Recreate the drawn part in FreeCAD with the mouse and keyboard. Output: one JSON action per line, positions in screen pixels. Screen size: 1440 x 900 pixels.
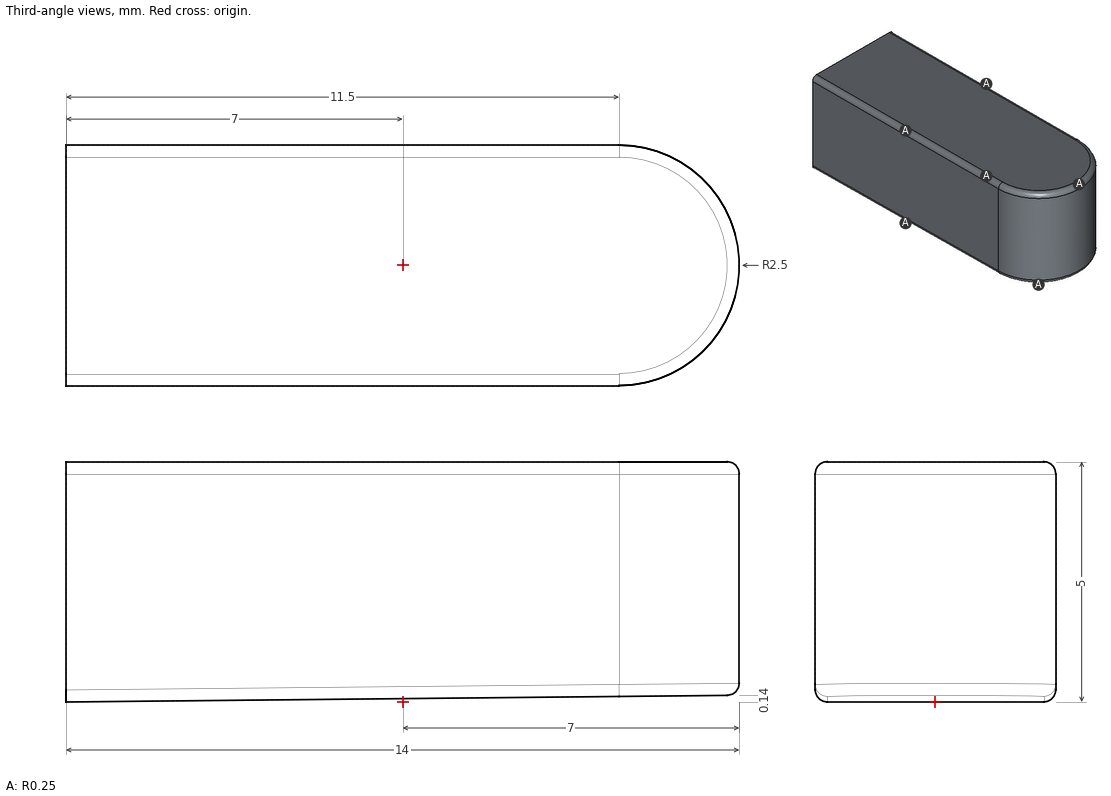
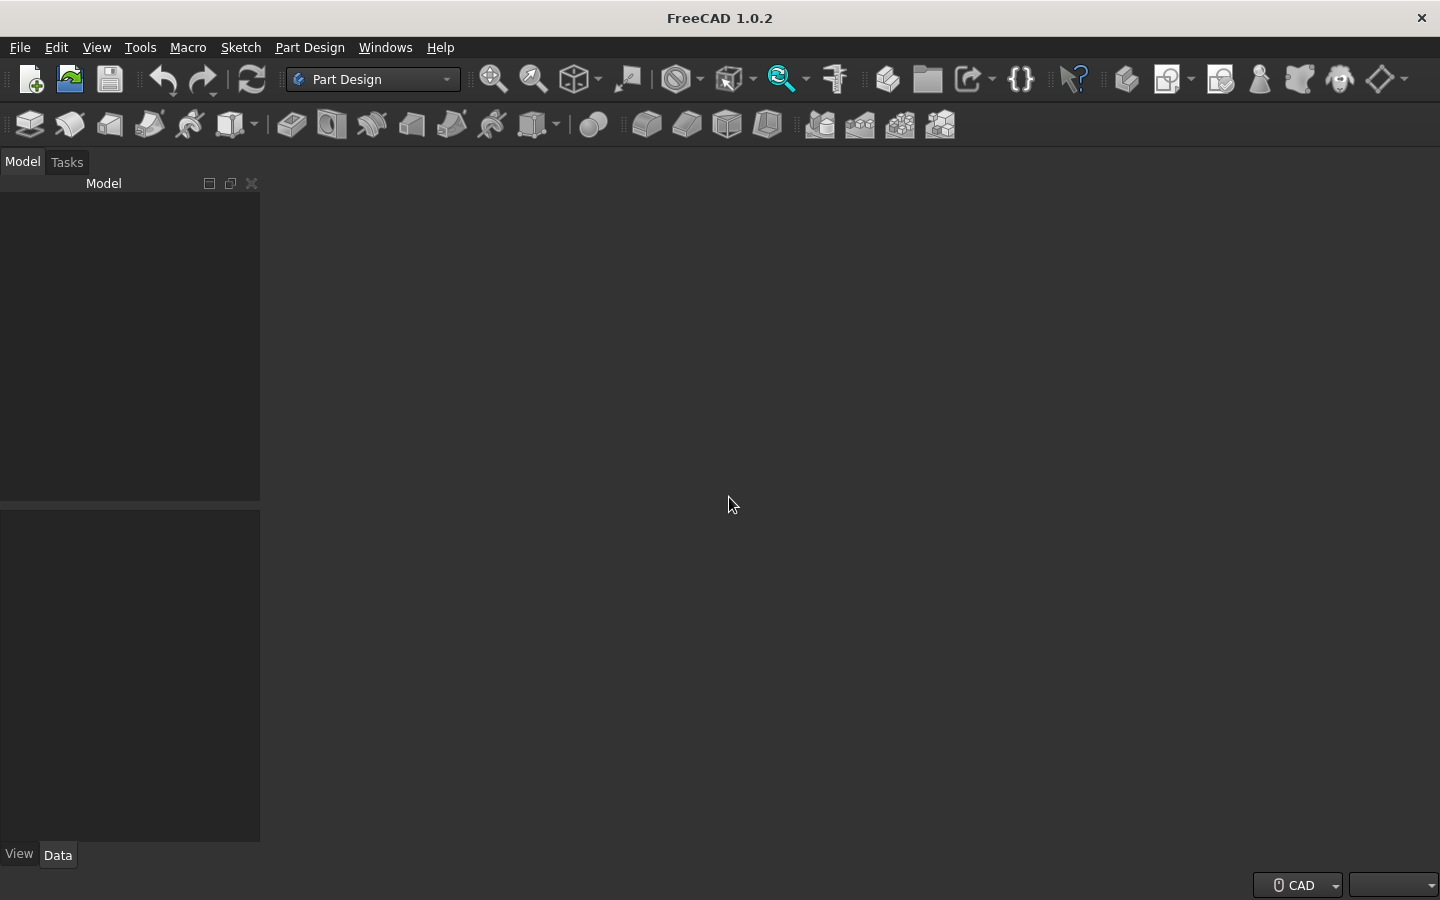
{"action": "key", "text": "ctrl+n"}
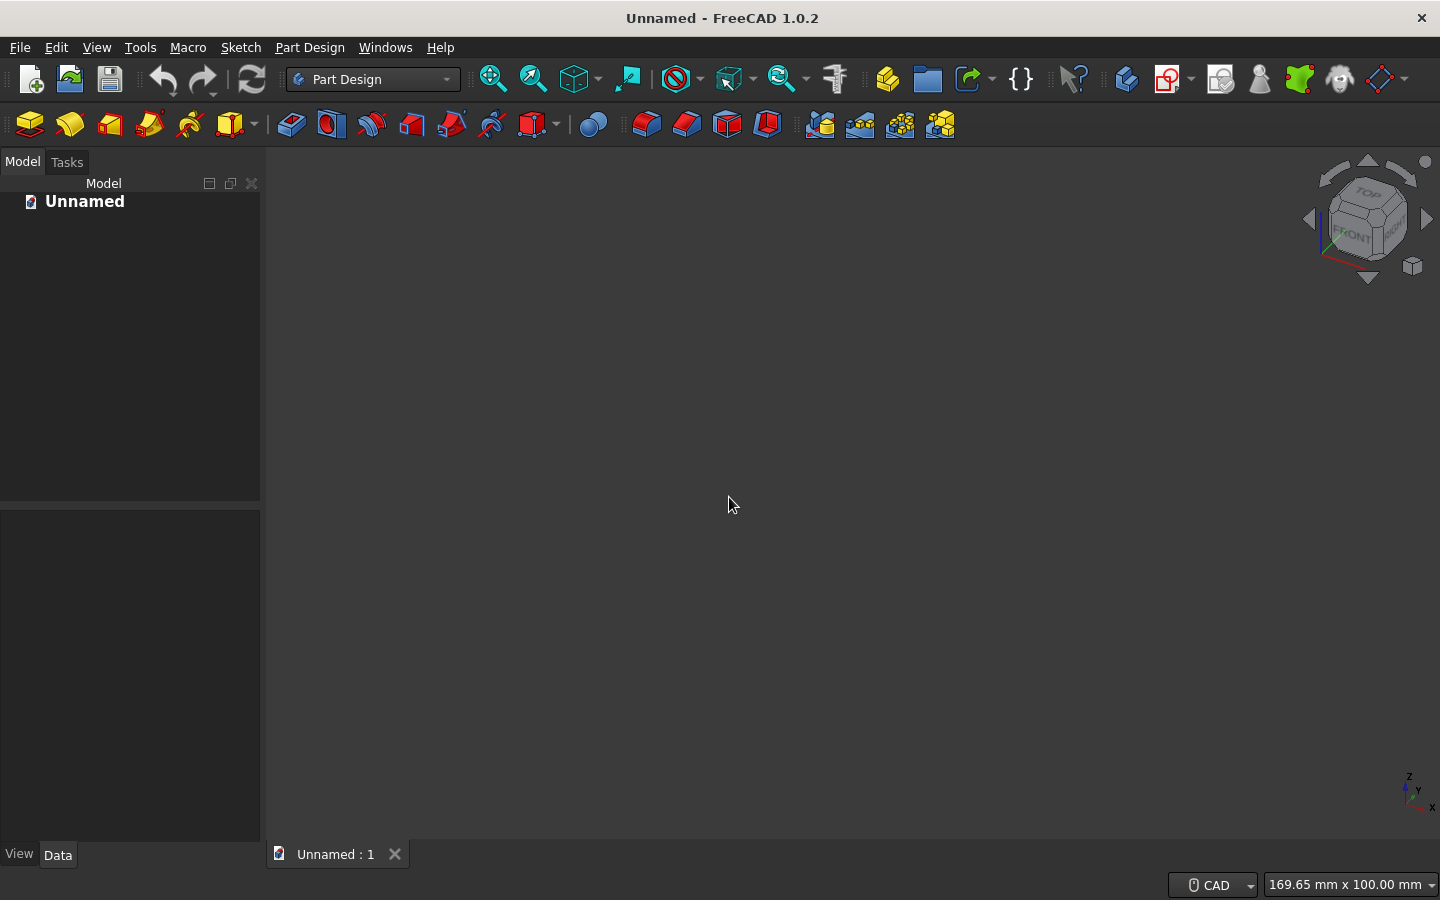
{"action": "left_click", "coordinate": [1168, 80]}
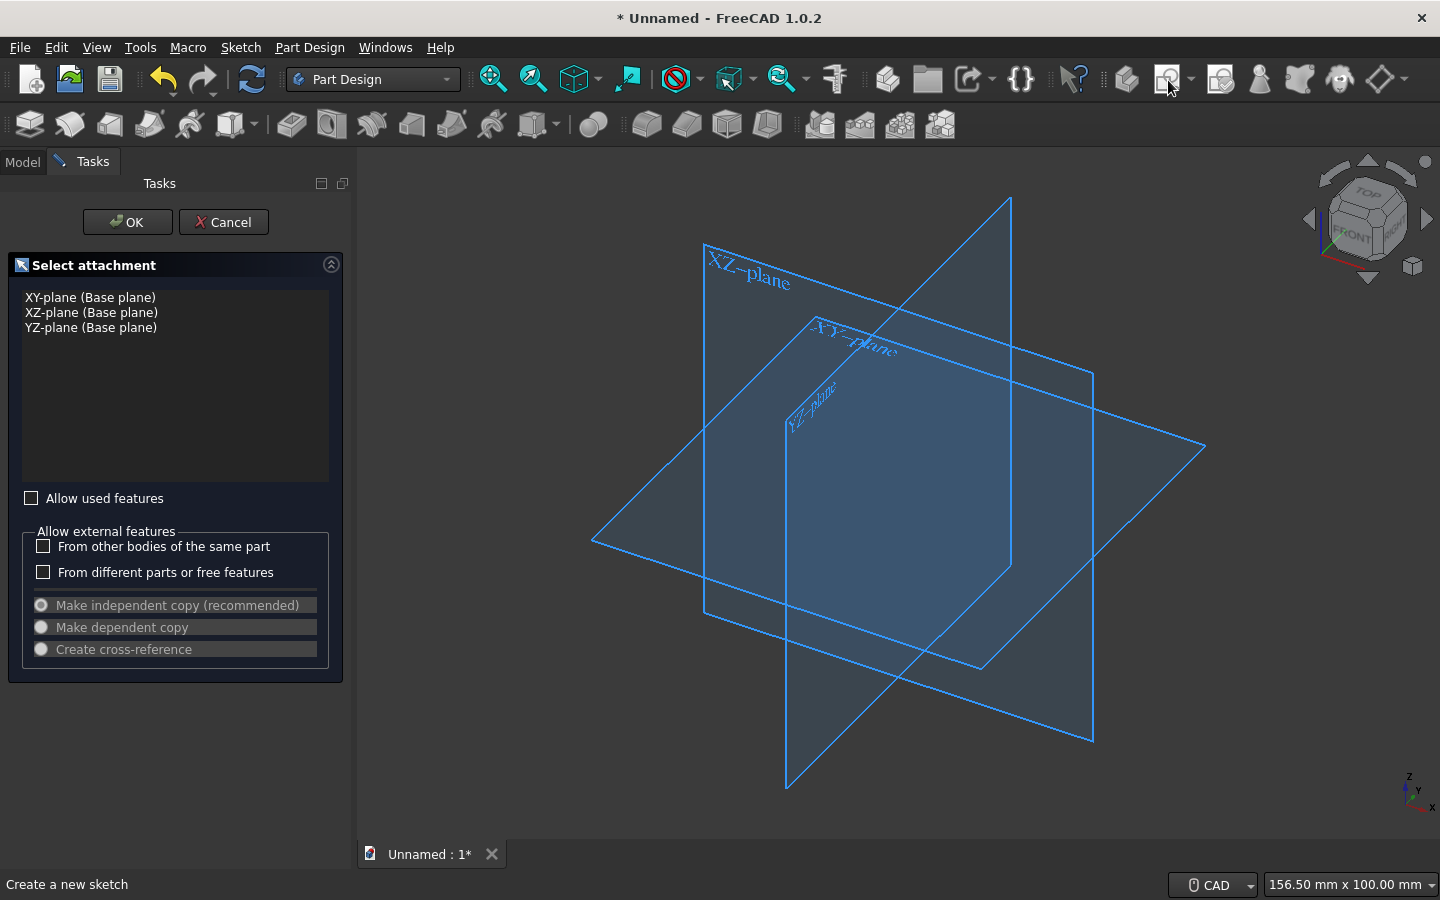
{"action": "left_click", "coordinate": [82, 298]}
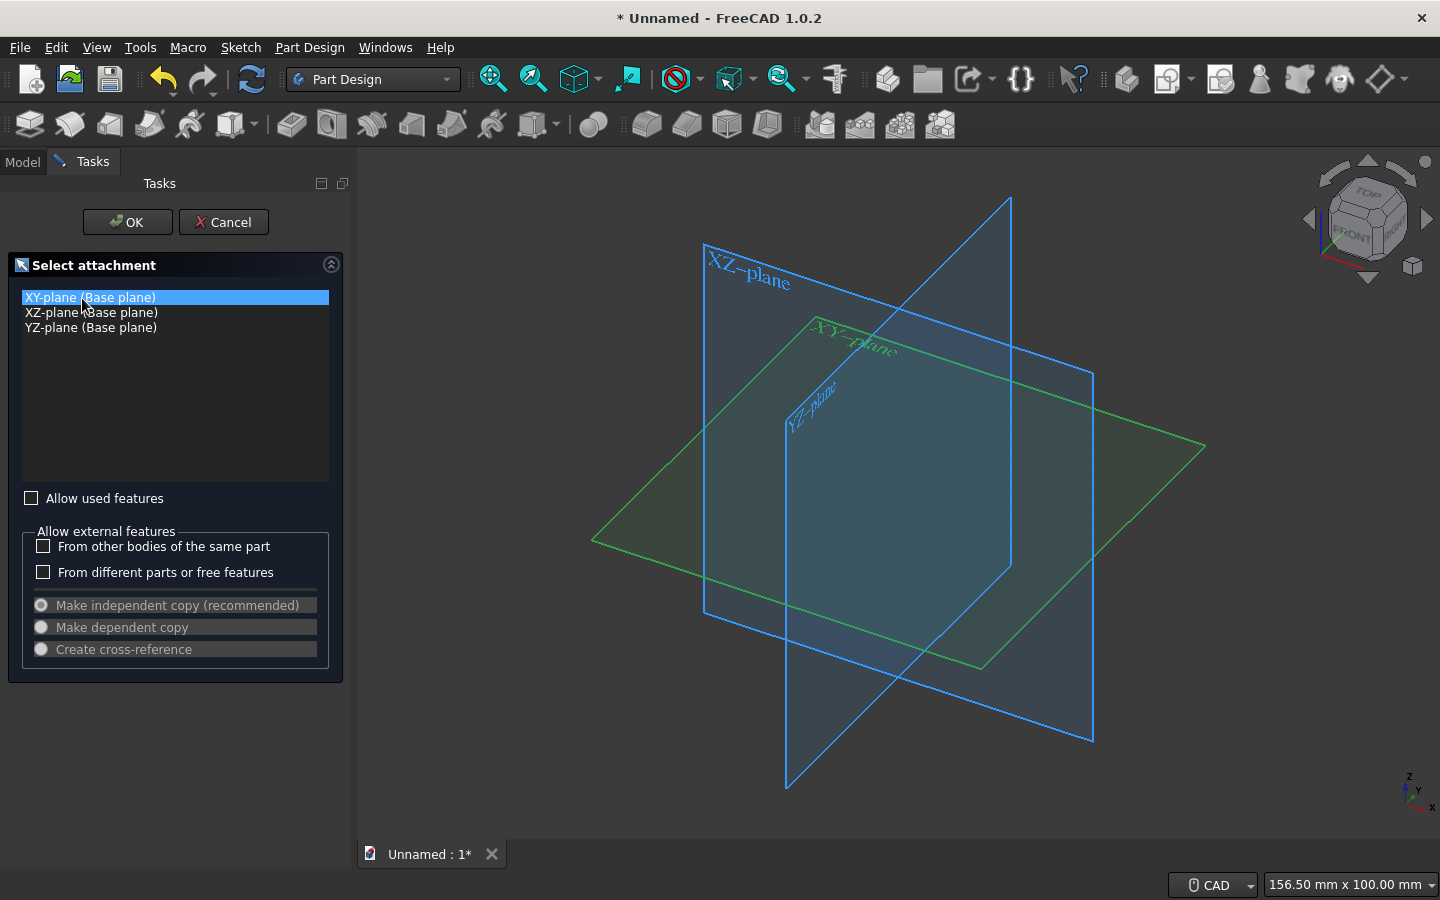
{"action": "left_click", "coordinate": [128, 222]}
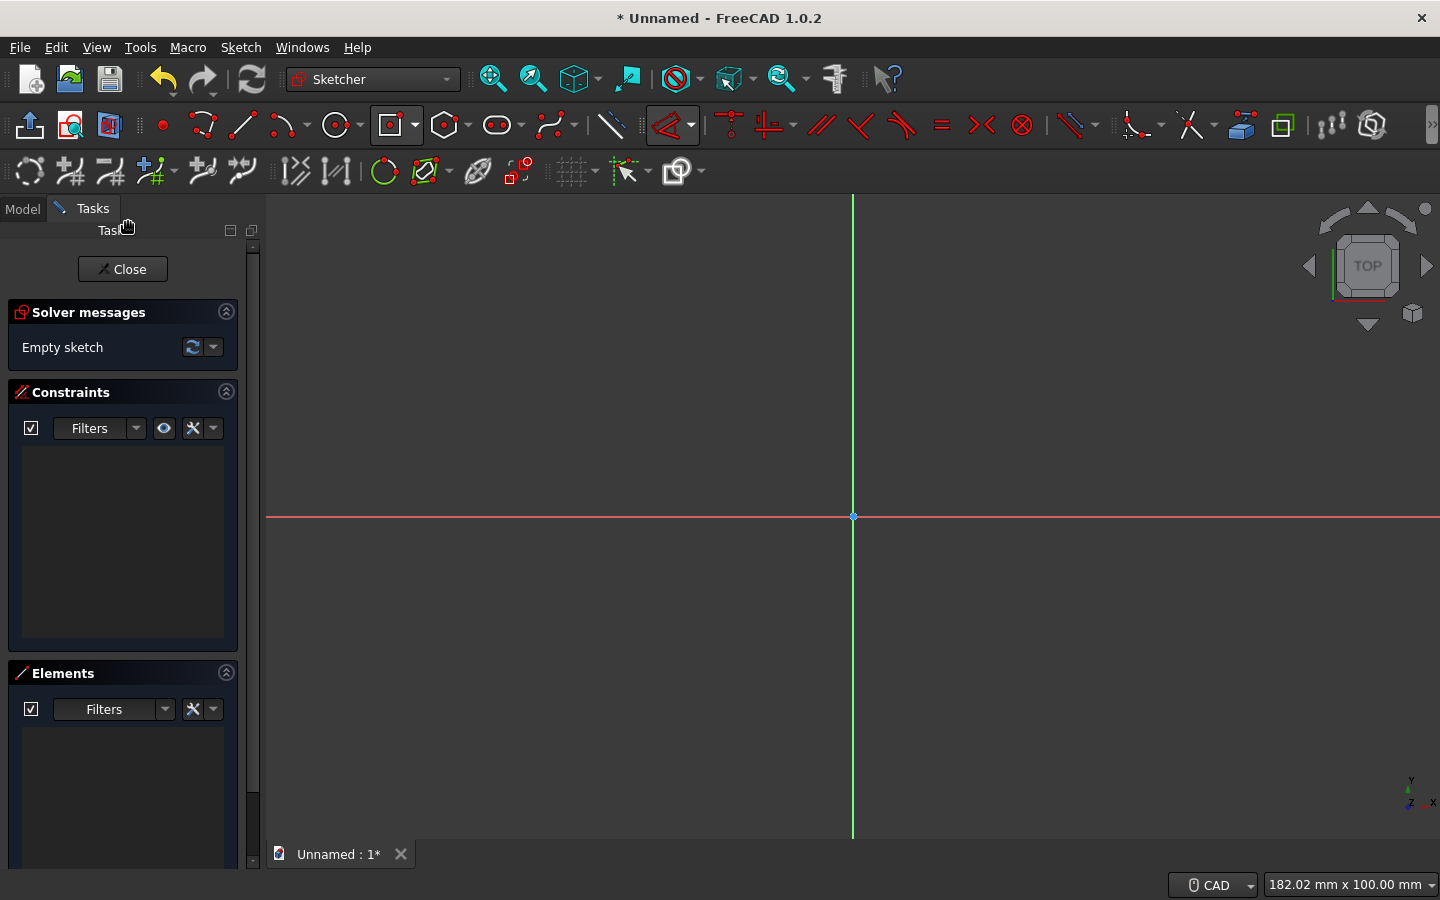
{"action": "scroll", "coordinate": [864, 516], "scroll_direction": "up", "scroll_amount": 10}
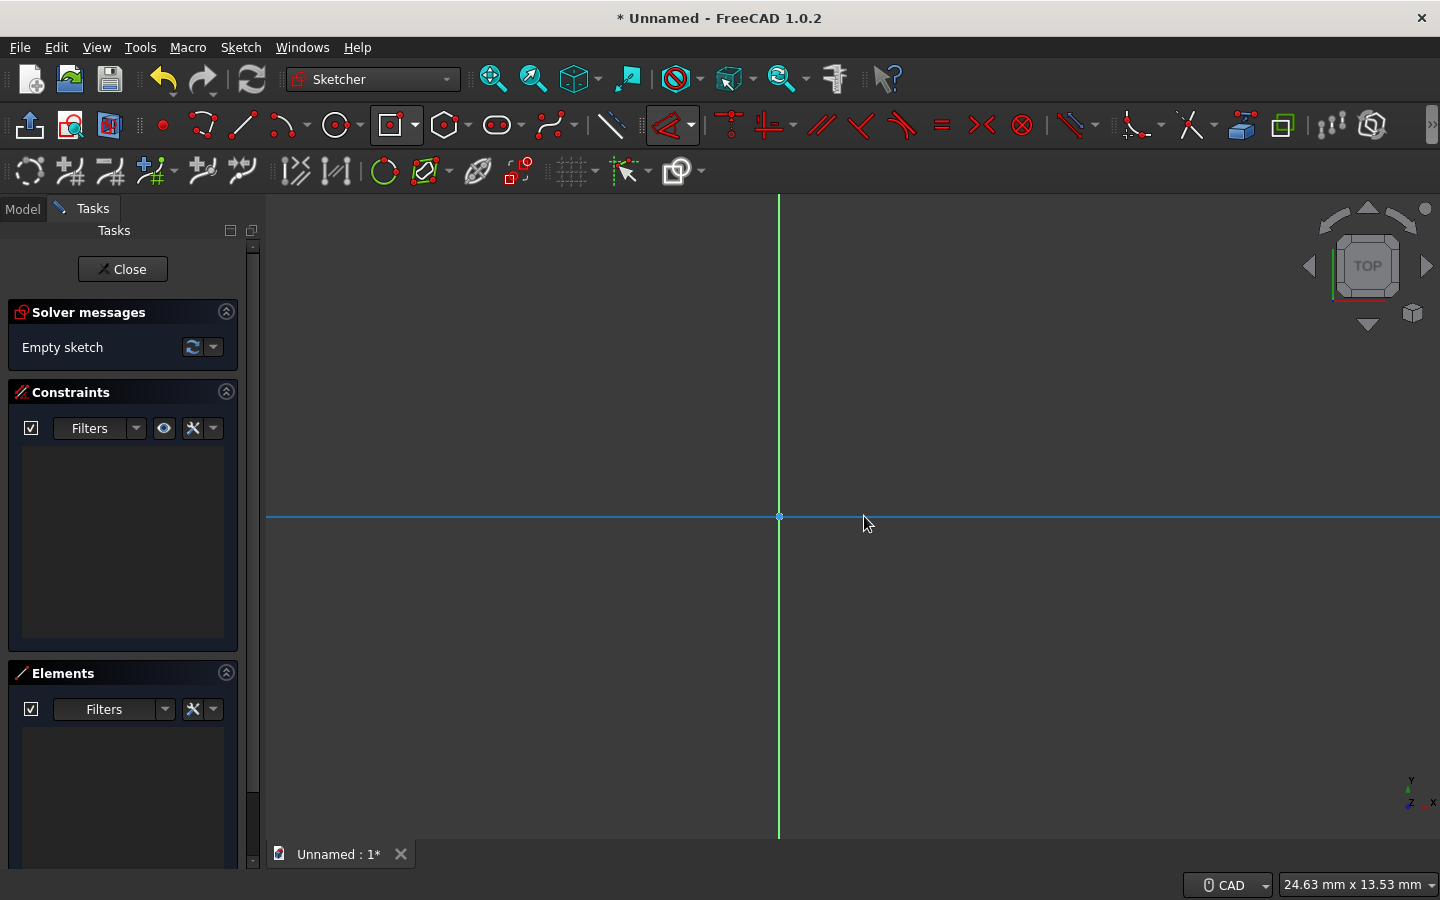
{"action": "key", "text": "g m"}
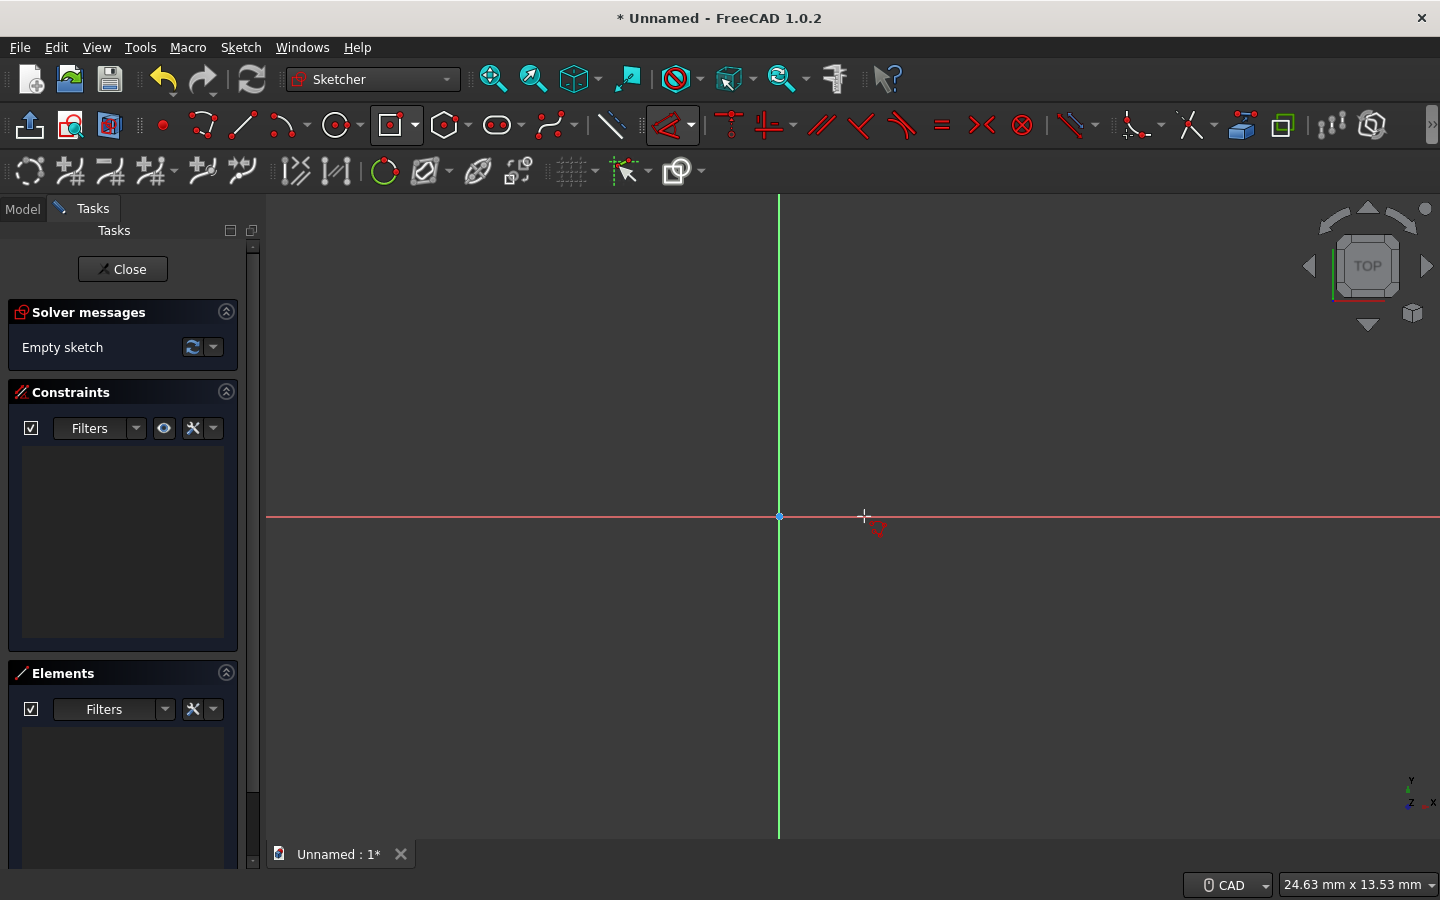
{"action": "left_click", "coordinate": [994, 397]}
{"action": "left_click", "coordinate": [446, 397]}
{"action": "left_click", "coordinate": [446, 636]}
{"action": "left_click", "coordinate": [994, 636]}
{"action": "right_click", "coordinate": [994, 636]}